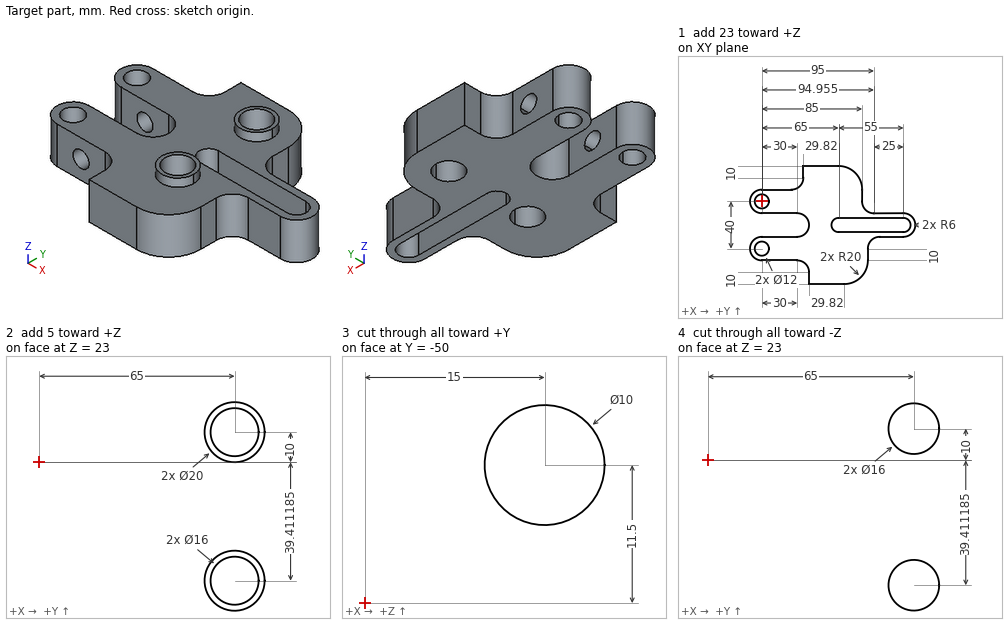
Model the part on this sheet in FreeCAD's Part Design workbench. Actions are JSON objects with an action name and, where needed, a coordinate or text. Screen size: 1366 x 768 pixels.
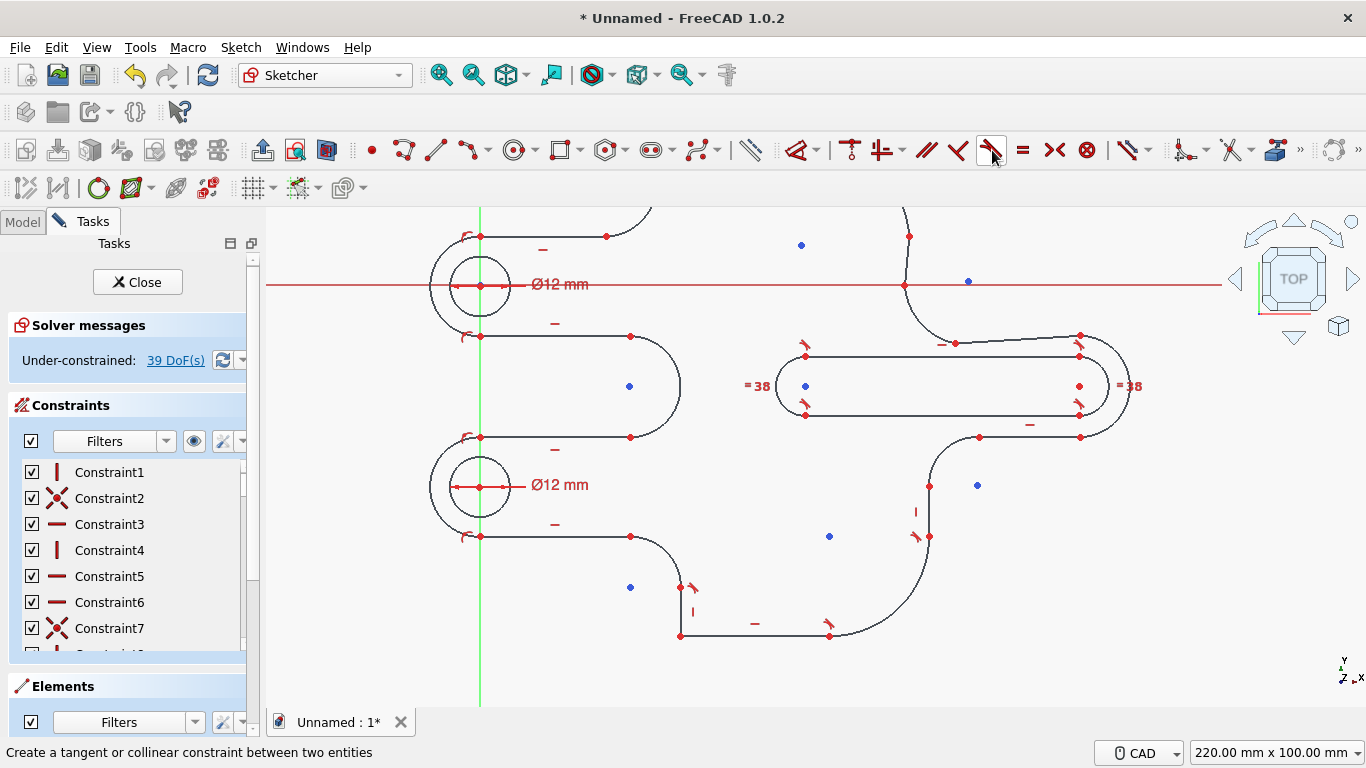
{"action": "left_click", "coordinate": [929, 522]}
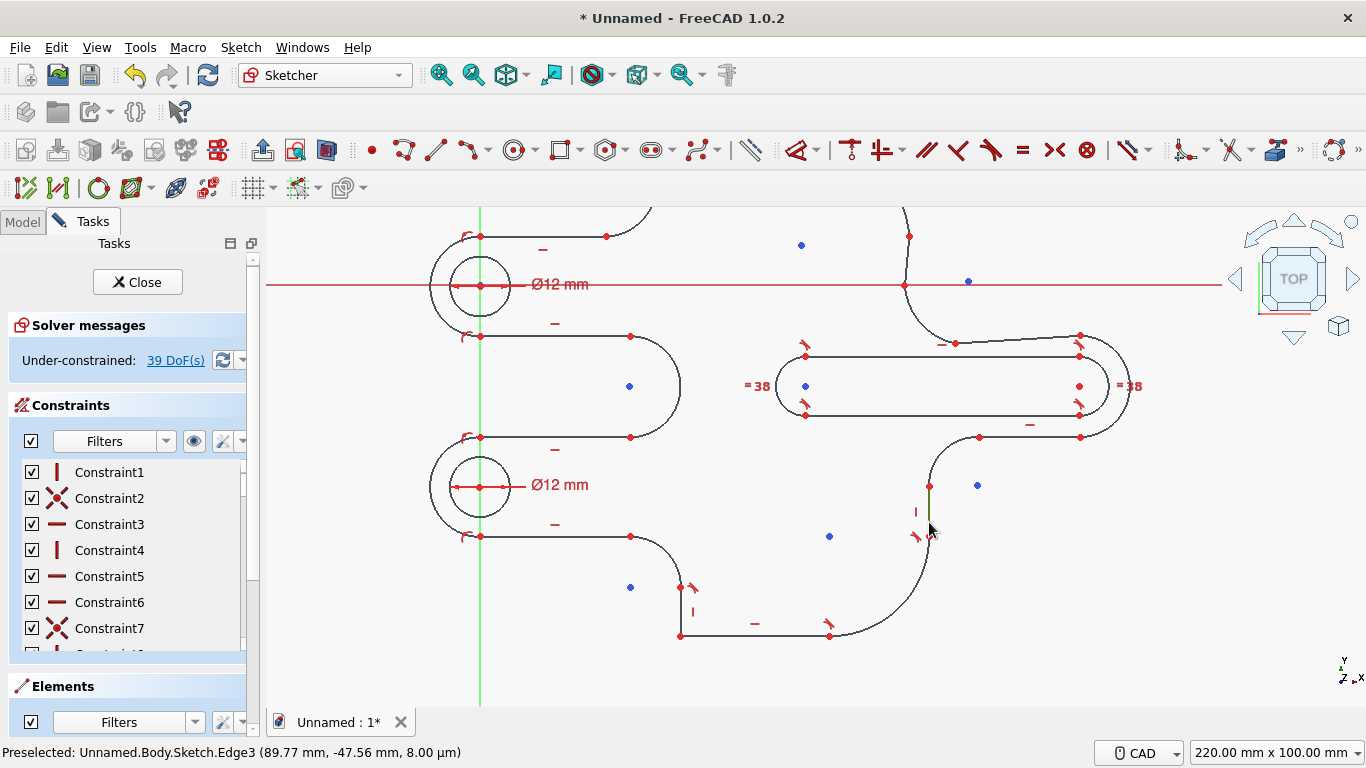
{"action": "left_click", "coordinate": [957, 442]}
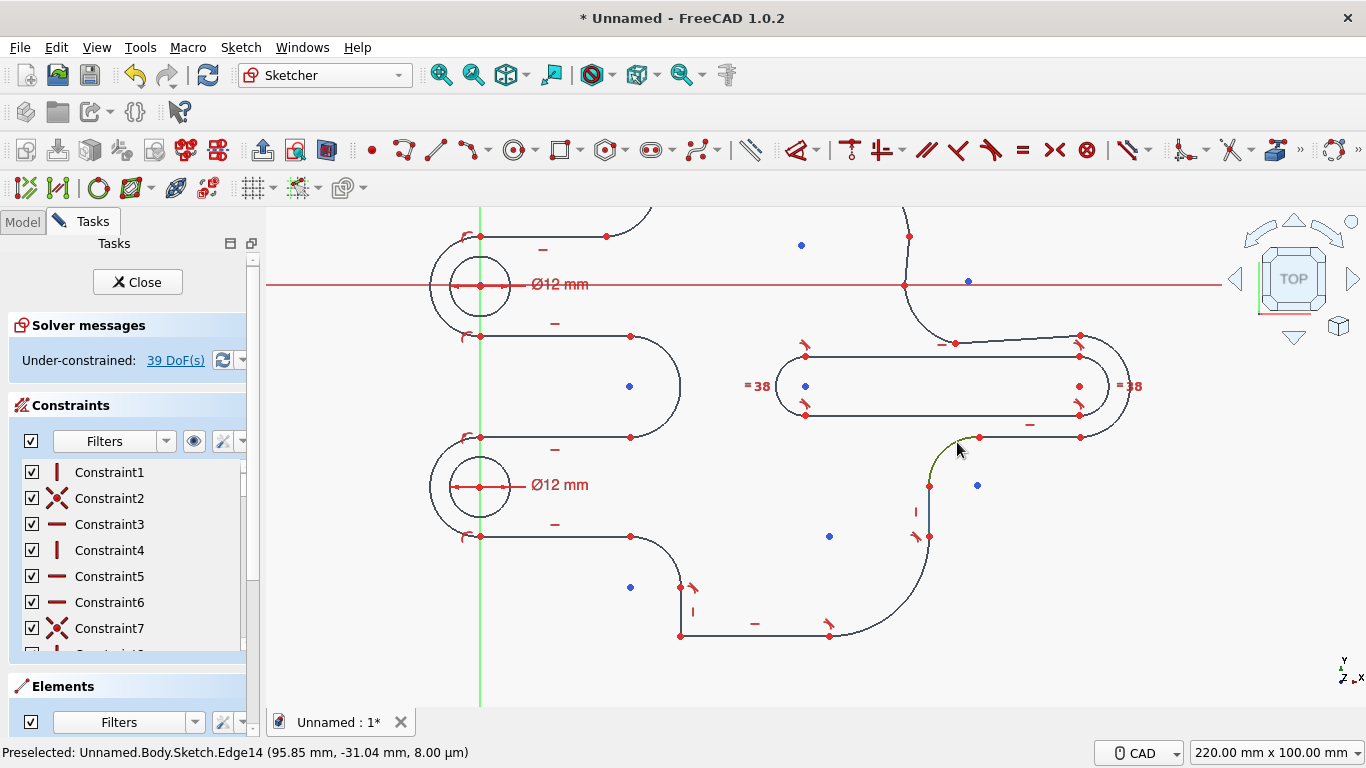
{"action": "left_click", "coordinate": [992, 150]}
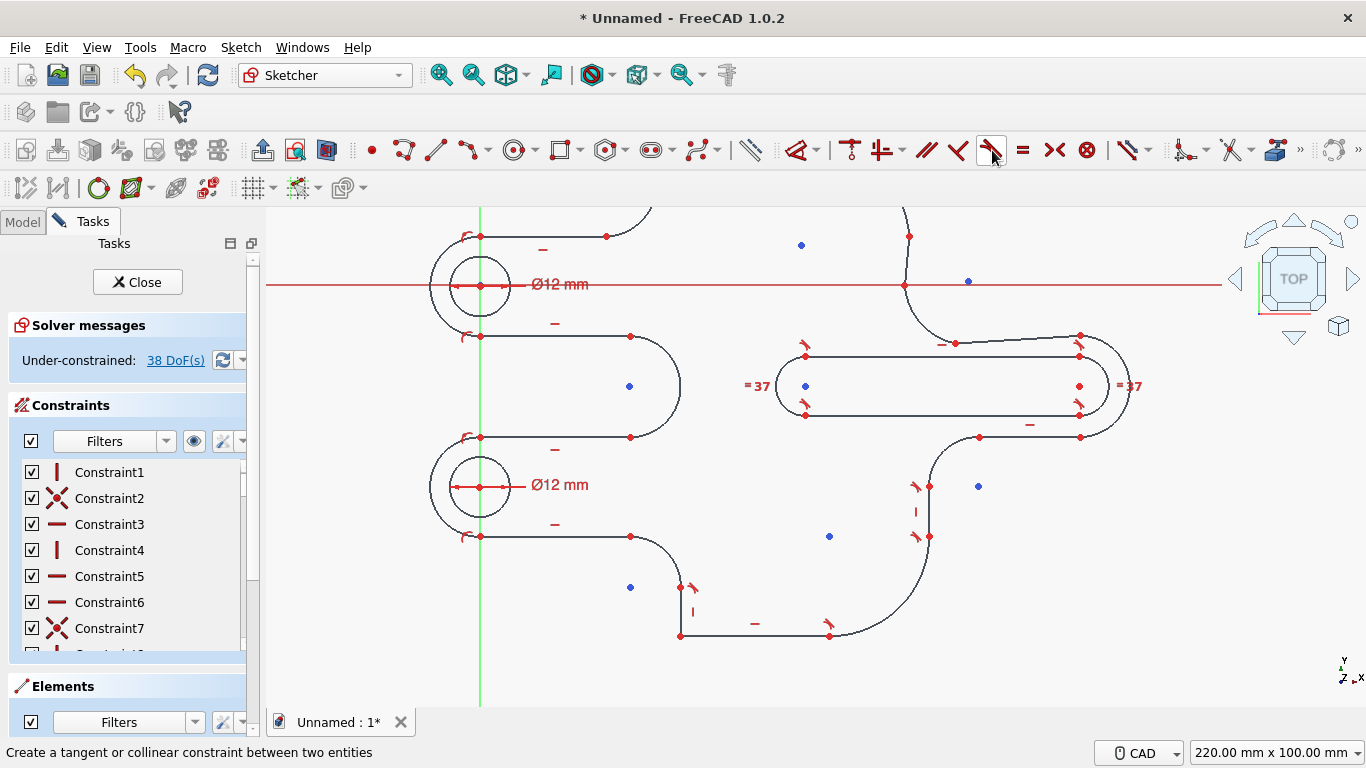
{"action": "left_click", "coordinate": [1010, 437]}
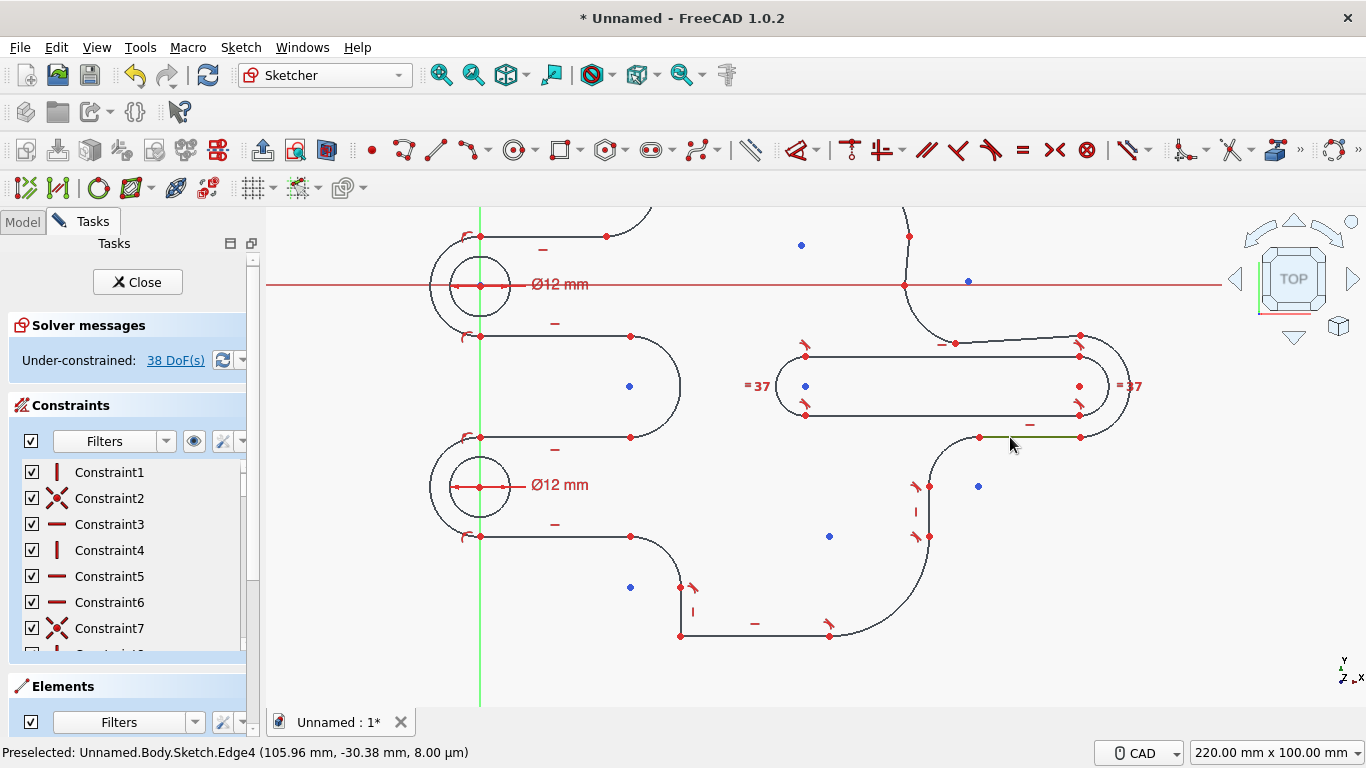
{"action": "left_click", "coordinate": [957, 442]}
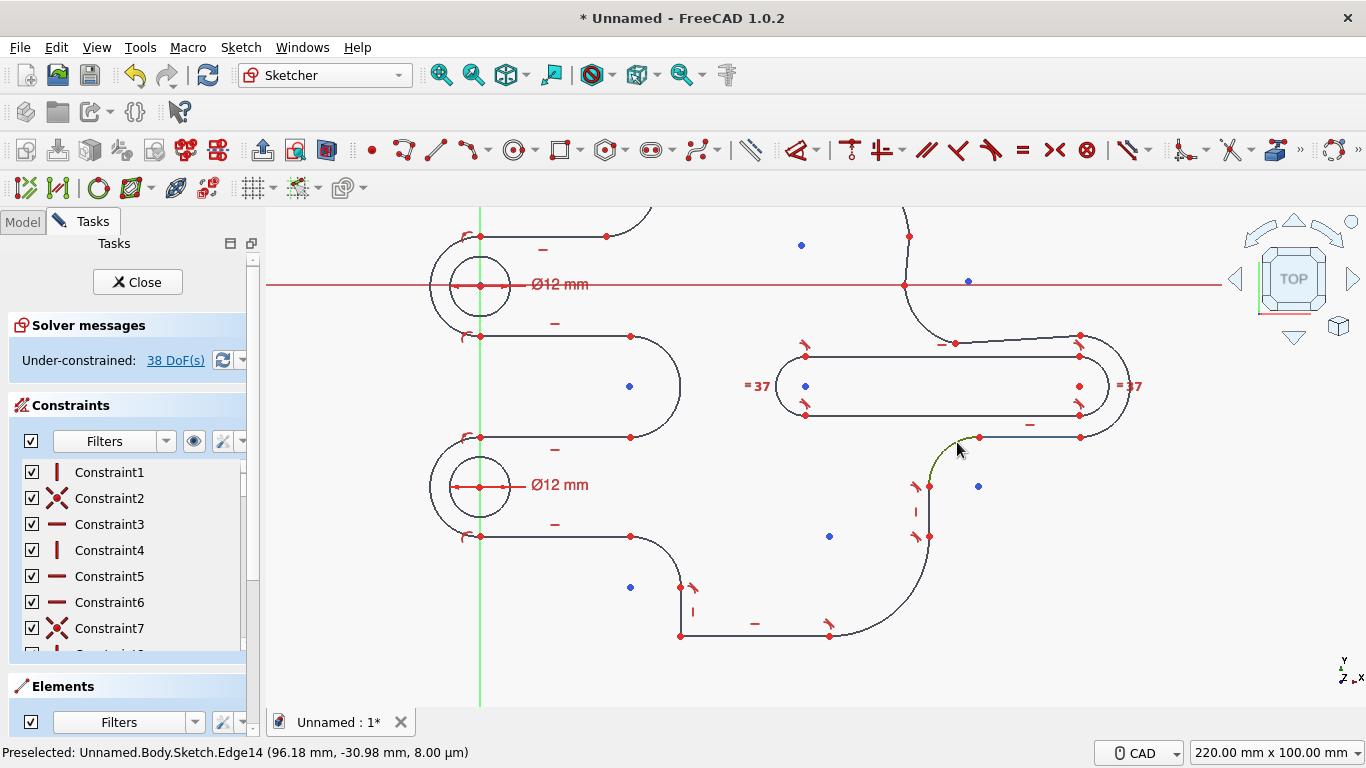
{"action": "left_click", "coordinate": [992, 150]}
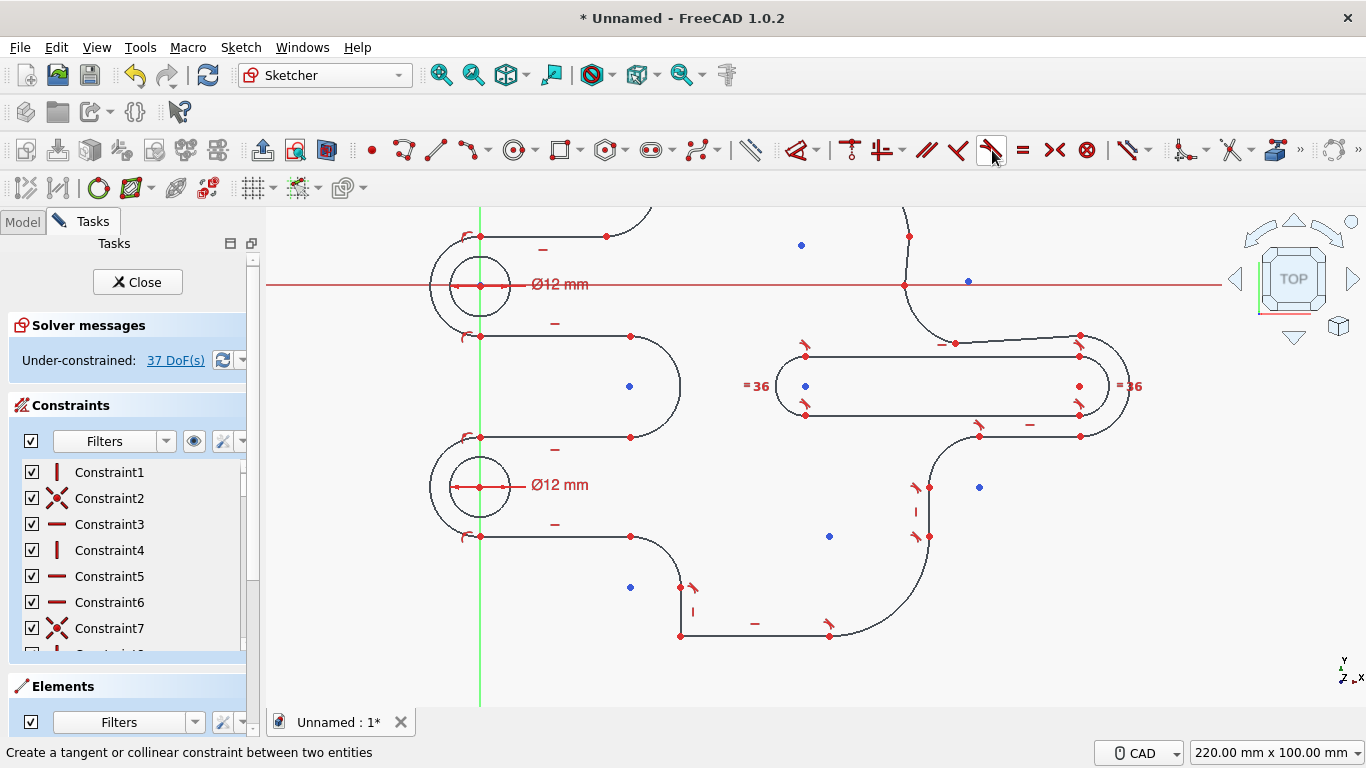
{"action": "left_click", "coordinate": [1010, 437]}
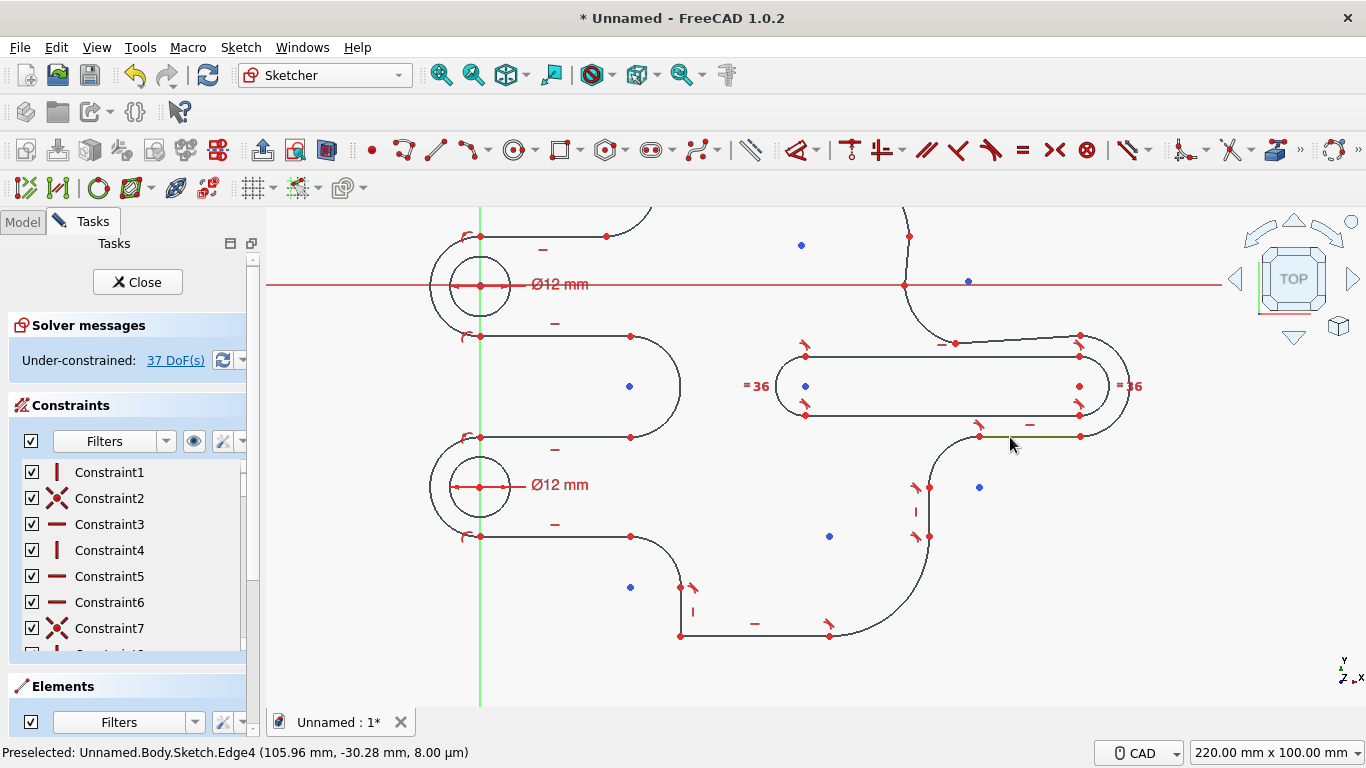
{"action": "left_click", "coordinate": [1120, 415]}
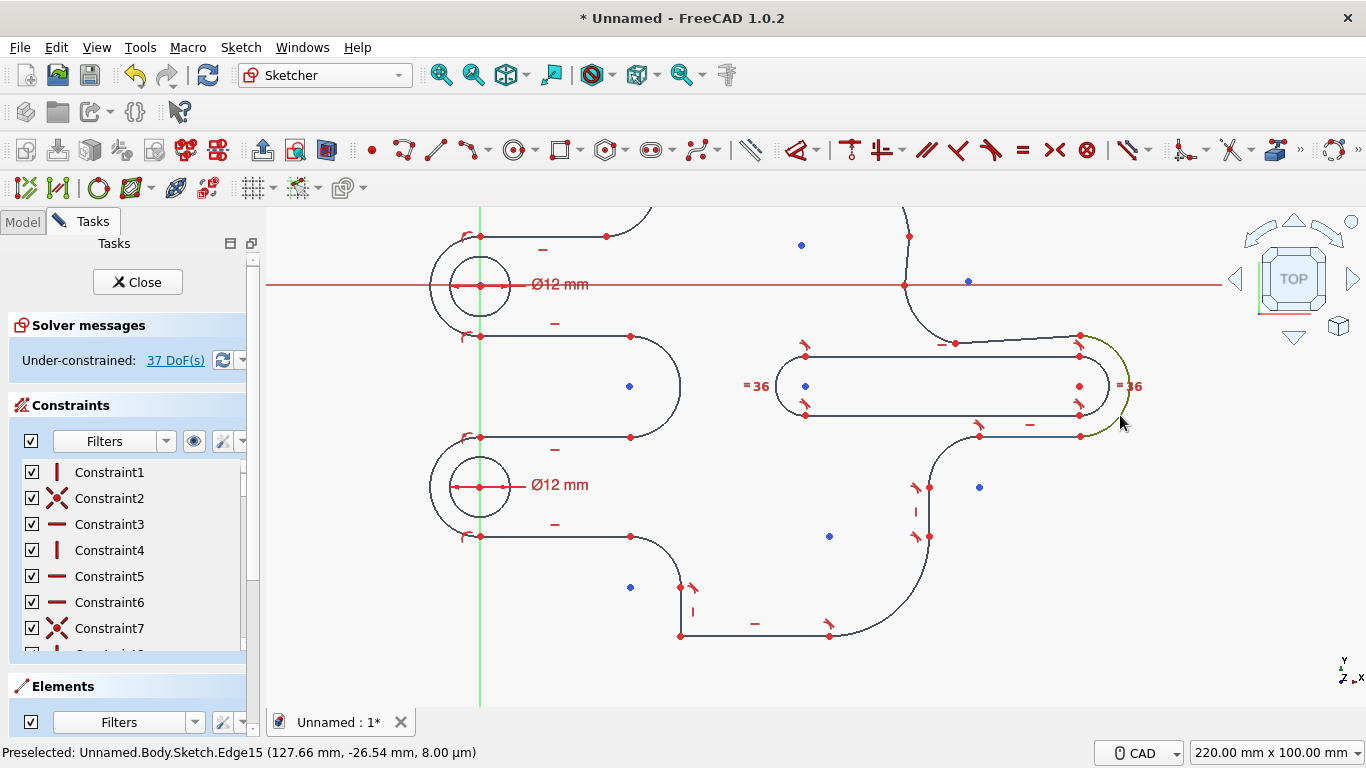
{"action": "left_click", "coordinate": [992, 150]}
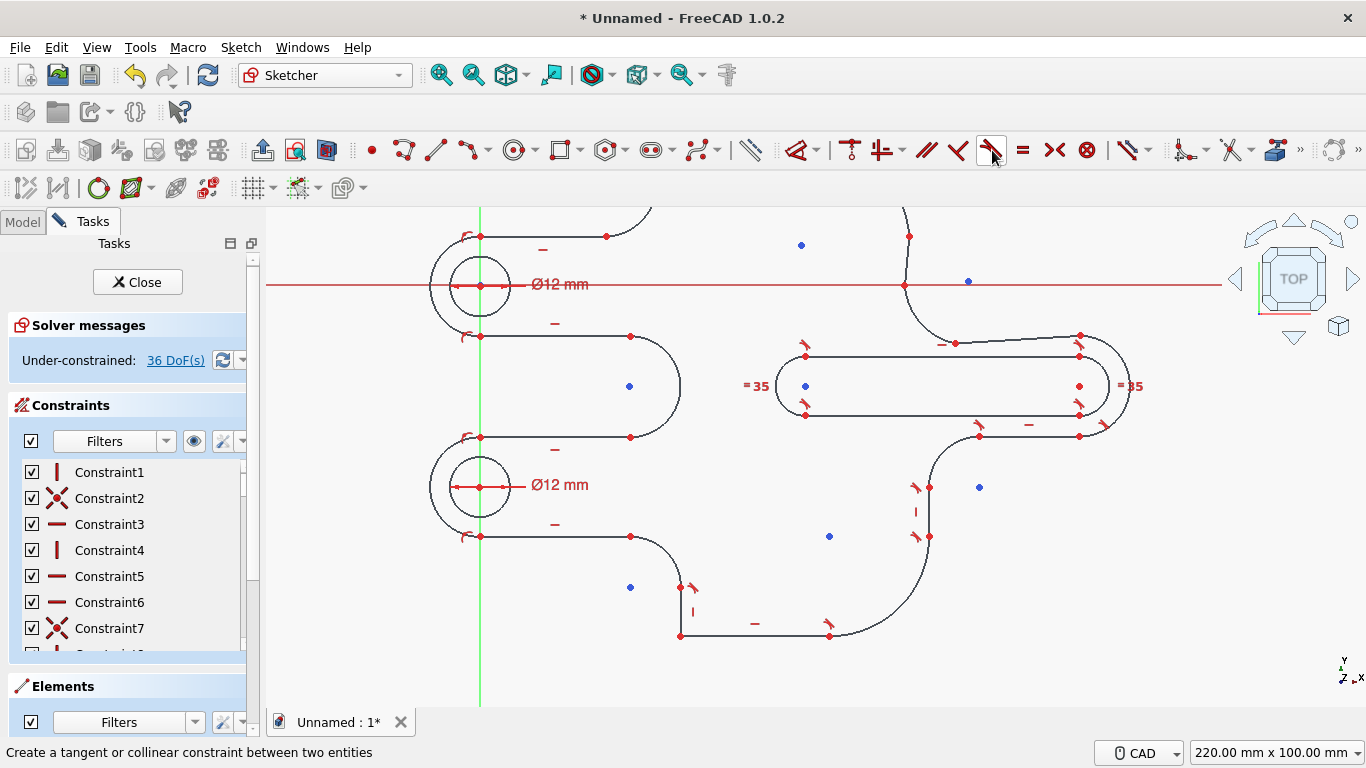
{"action": "left_click", "coordinate": [1043, 338]}